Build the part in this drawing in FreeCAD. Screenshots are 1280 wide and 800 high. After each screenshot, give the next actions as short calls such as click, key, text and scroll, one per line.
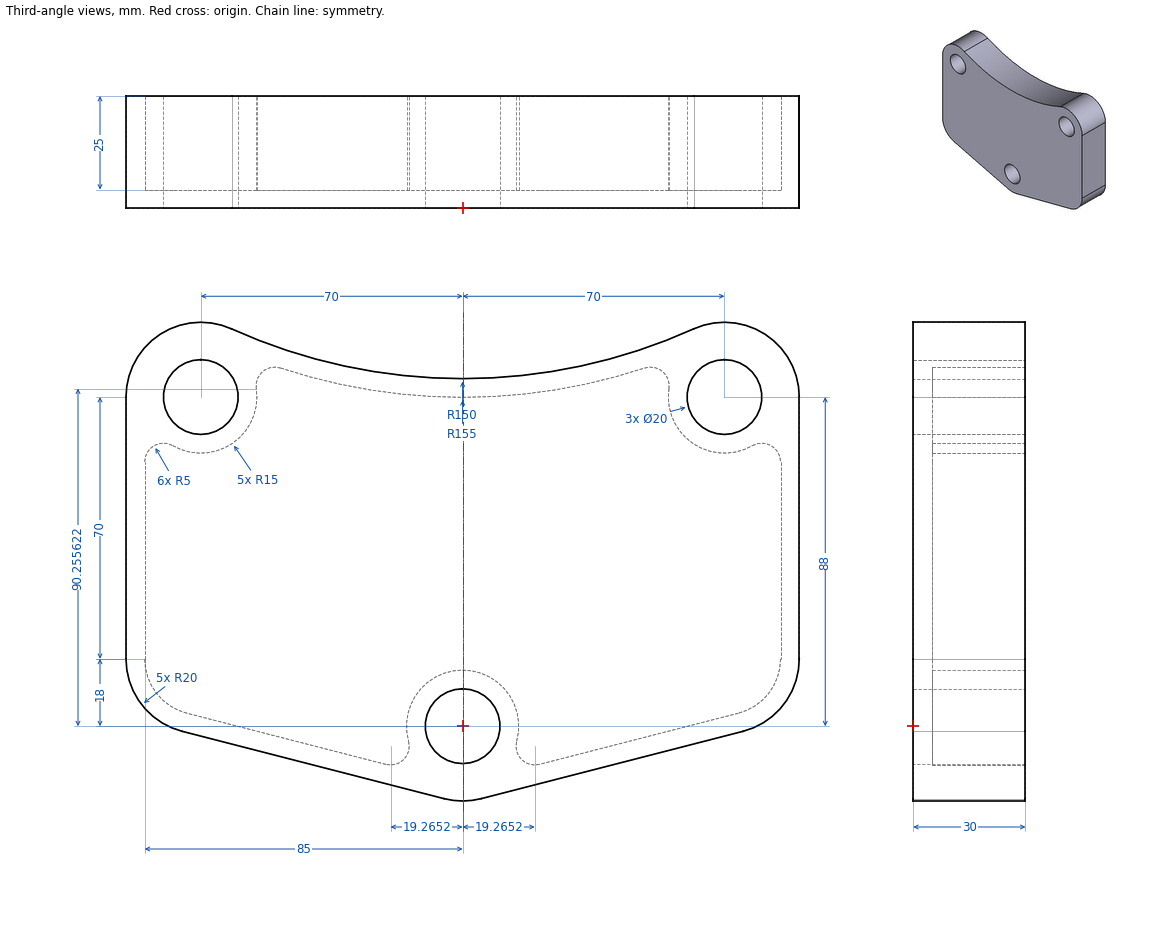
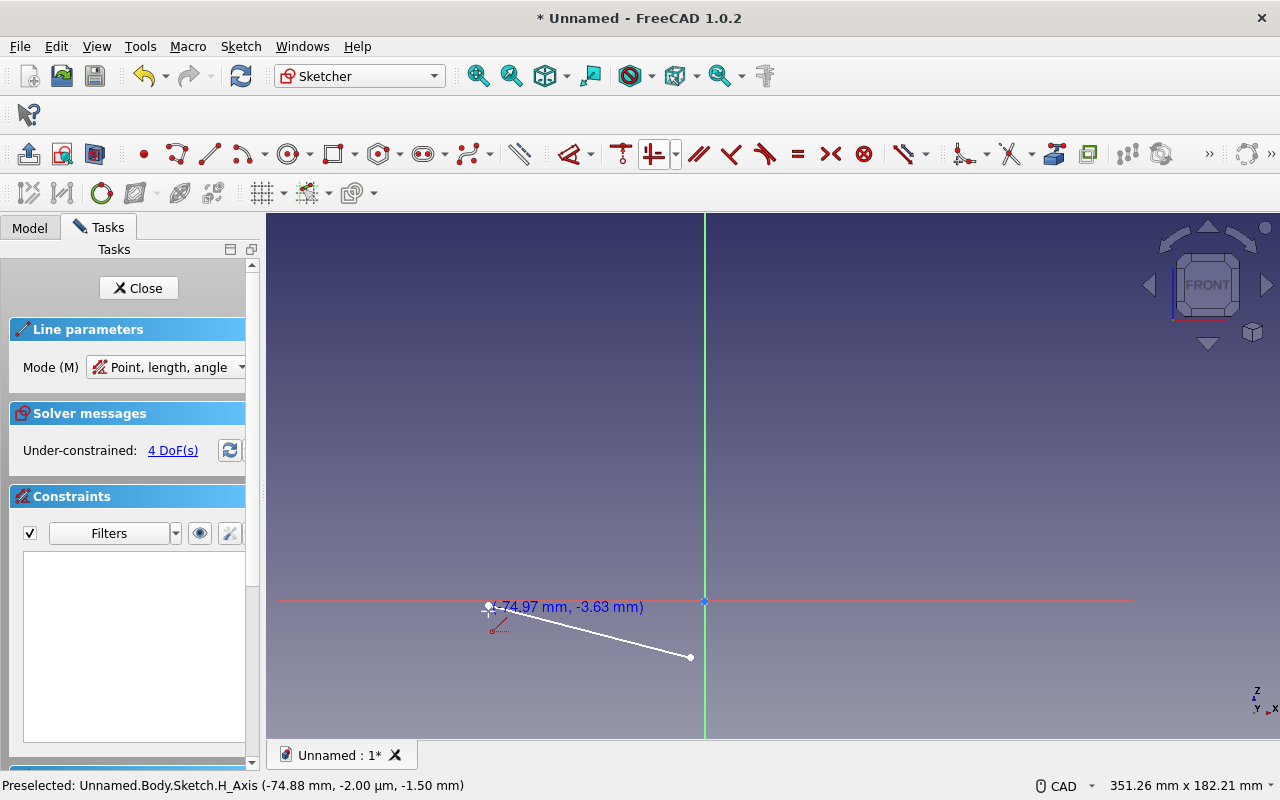
click(445, 549)
click(445, 347)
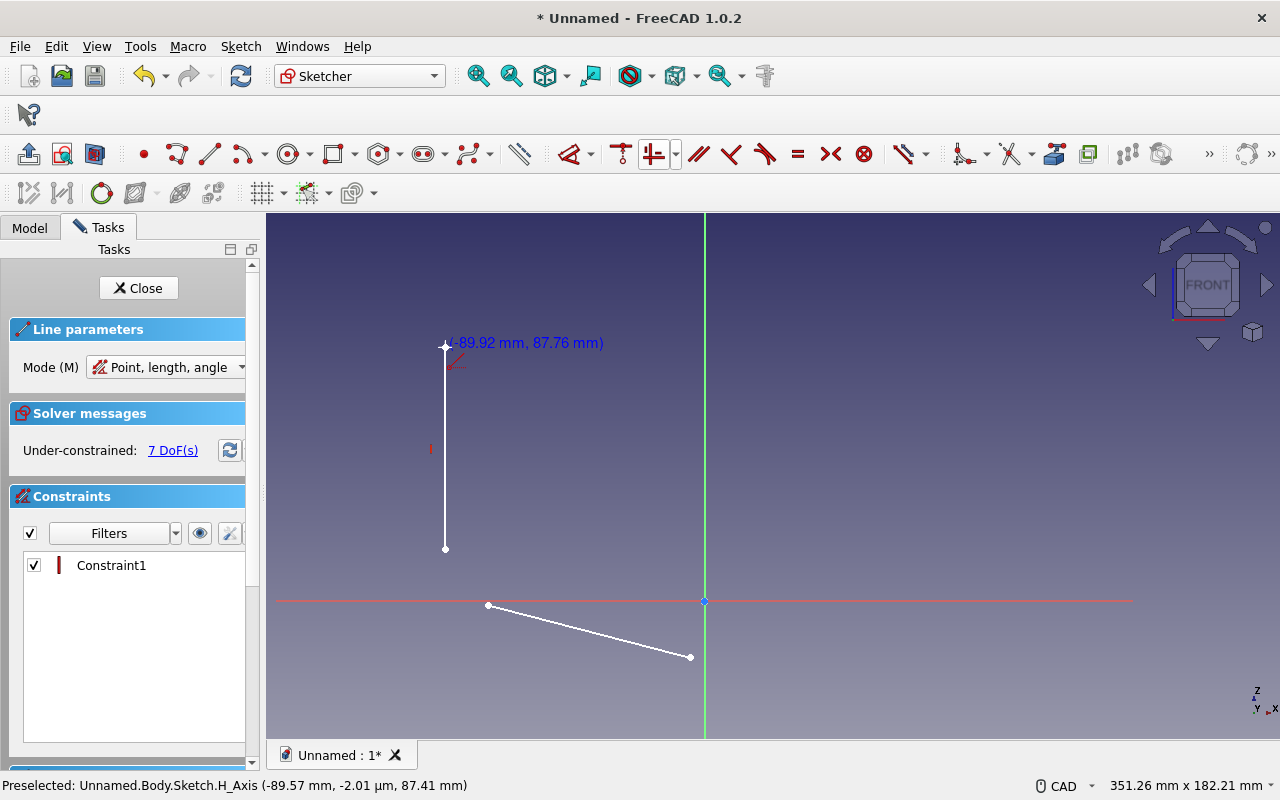
click(964, 347)
click(964, 549)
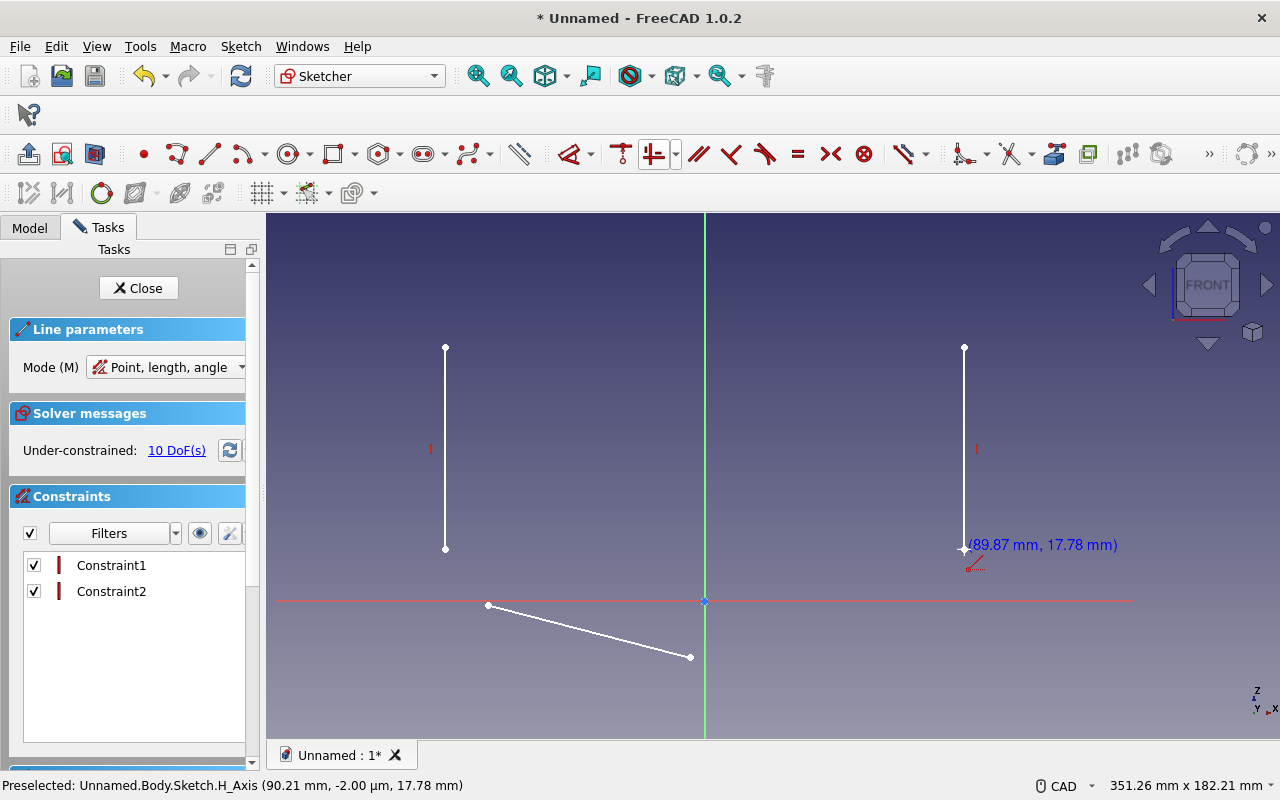
scroll(921, 605, up, 7)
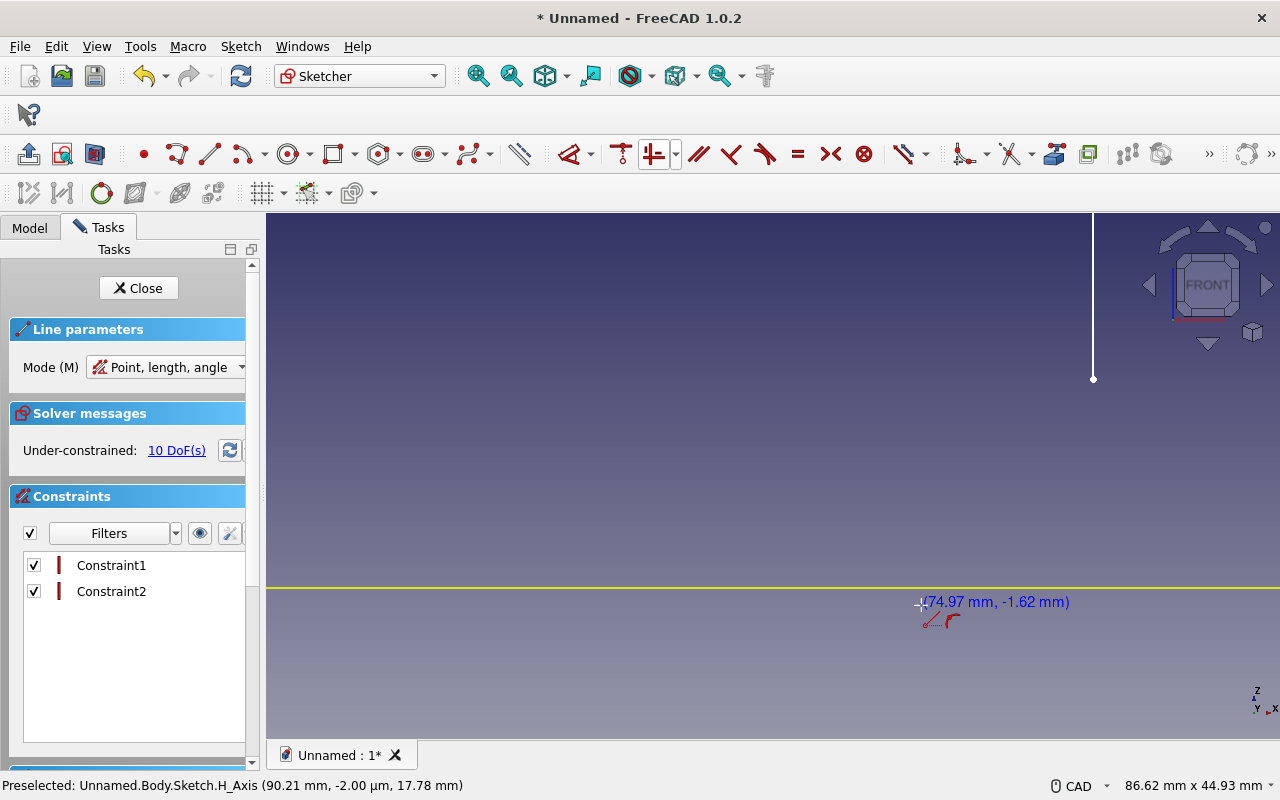
click(919, 604)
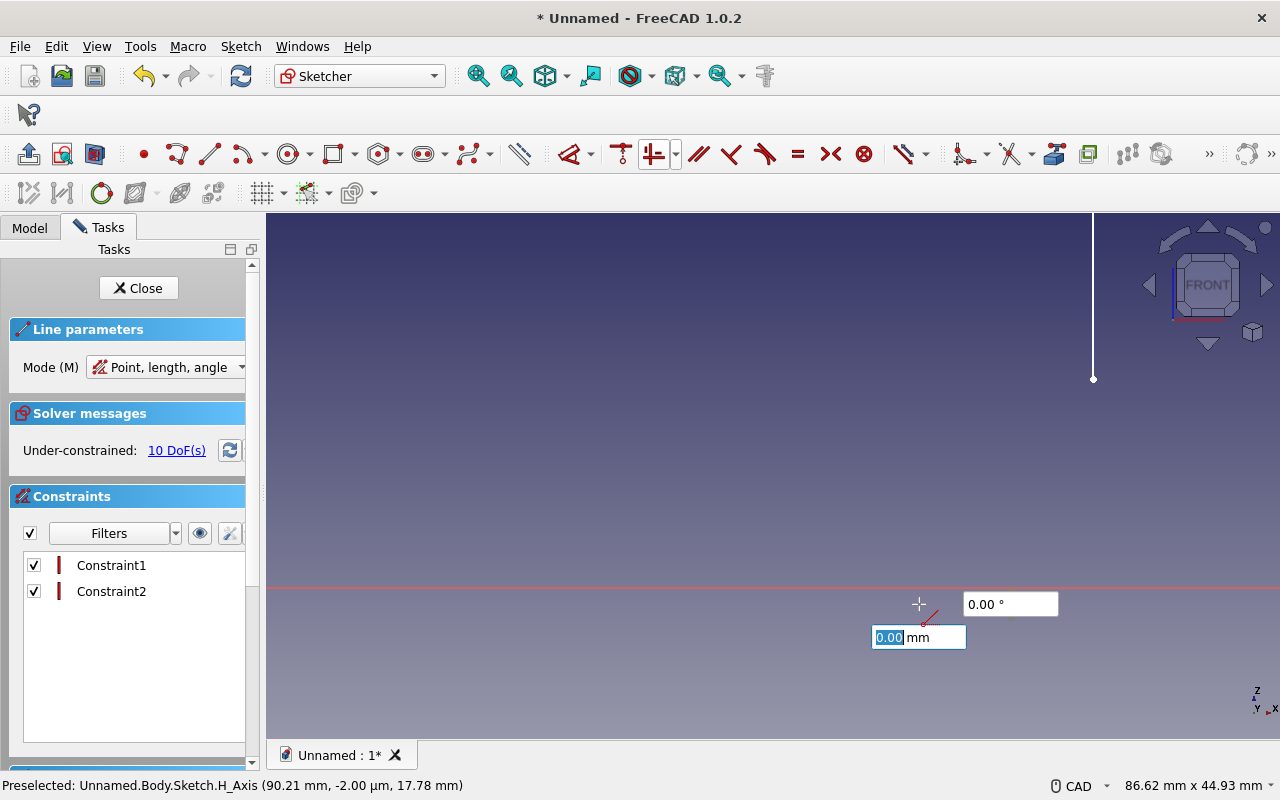
scroll(922, 605, down, 7)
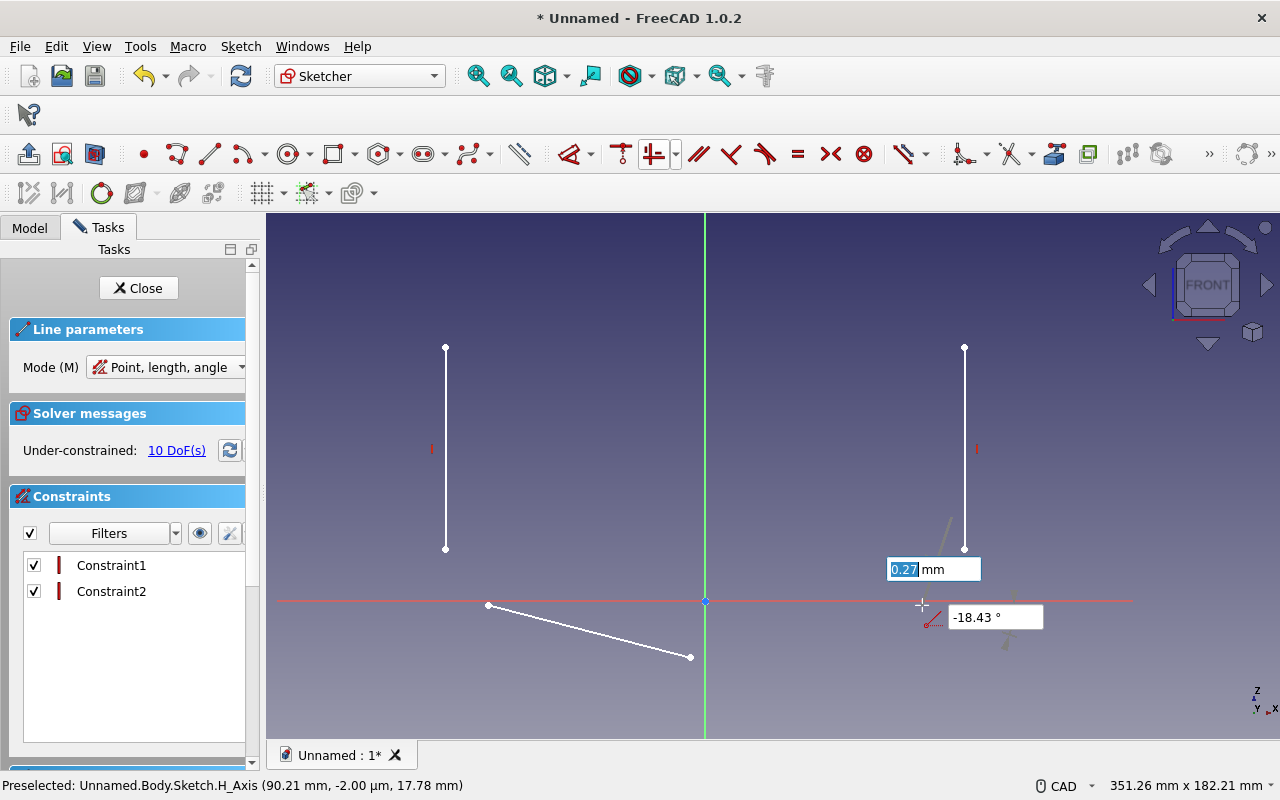
click(720, 657)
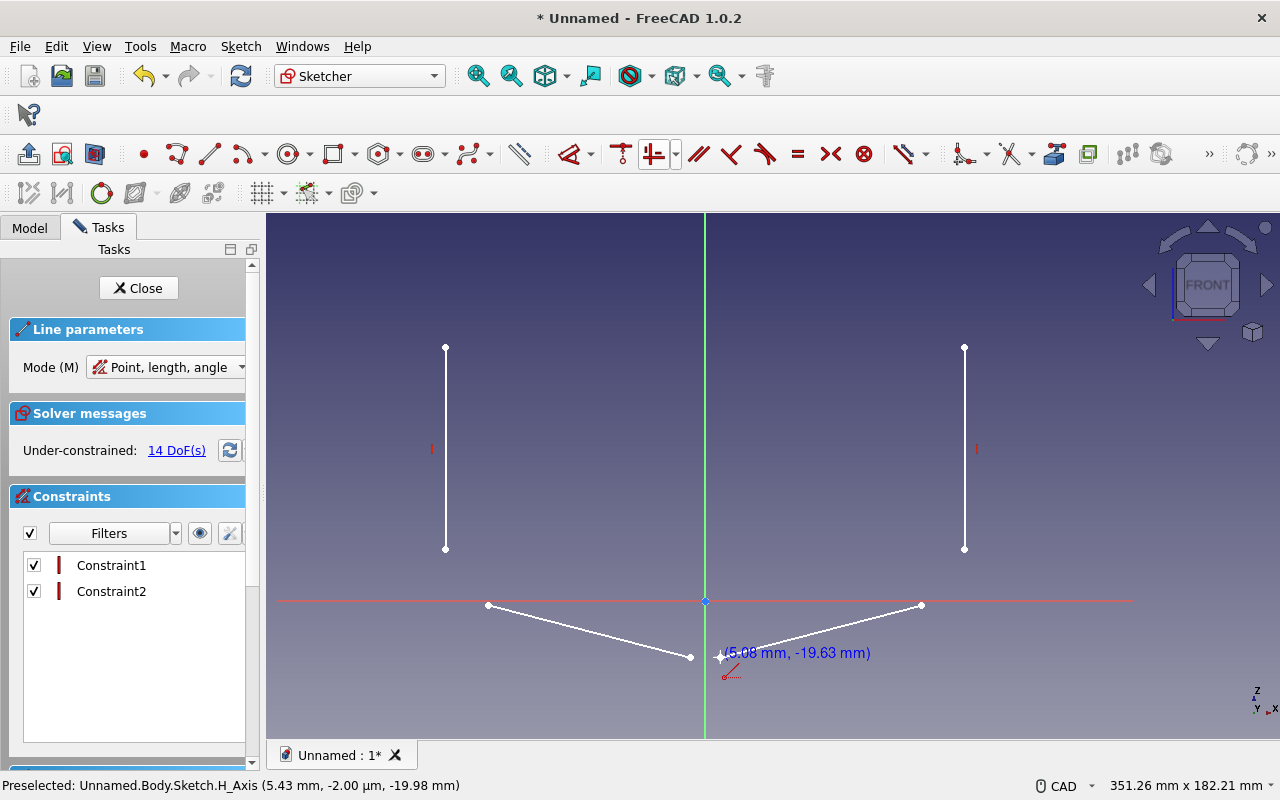
key(g)
key(3)
key(a)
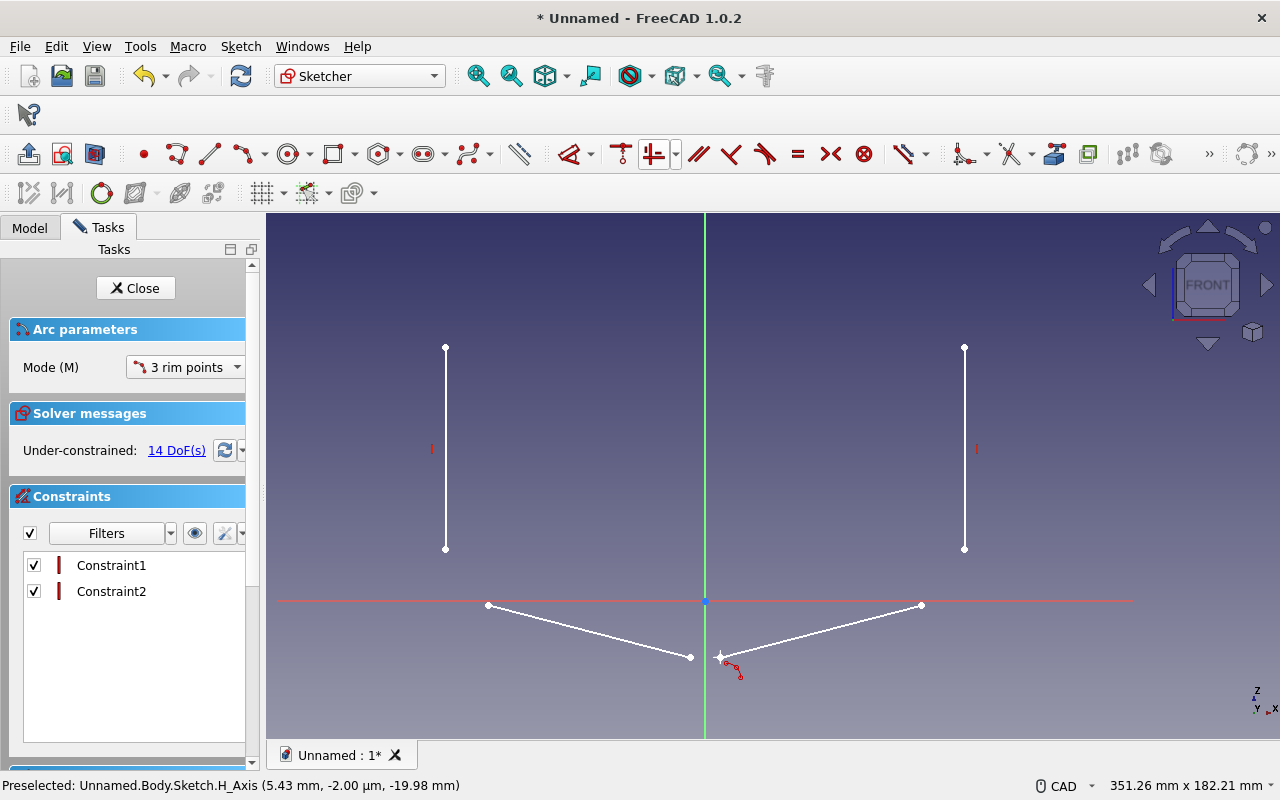
scroll(489, 605, up, 7)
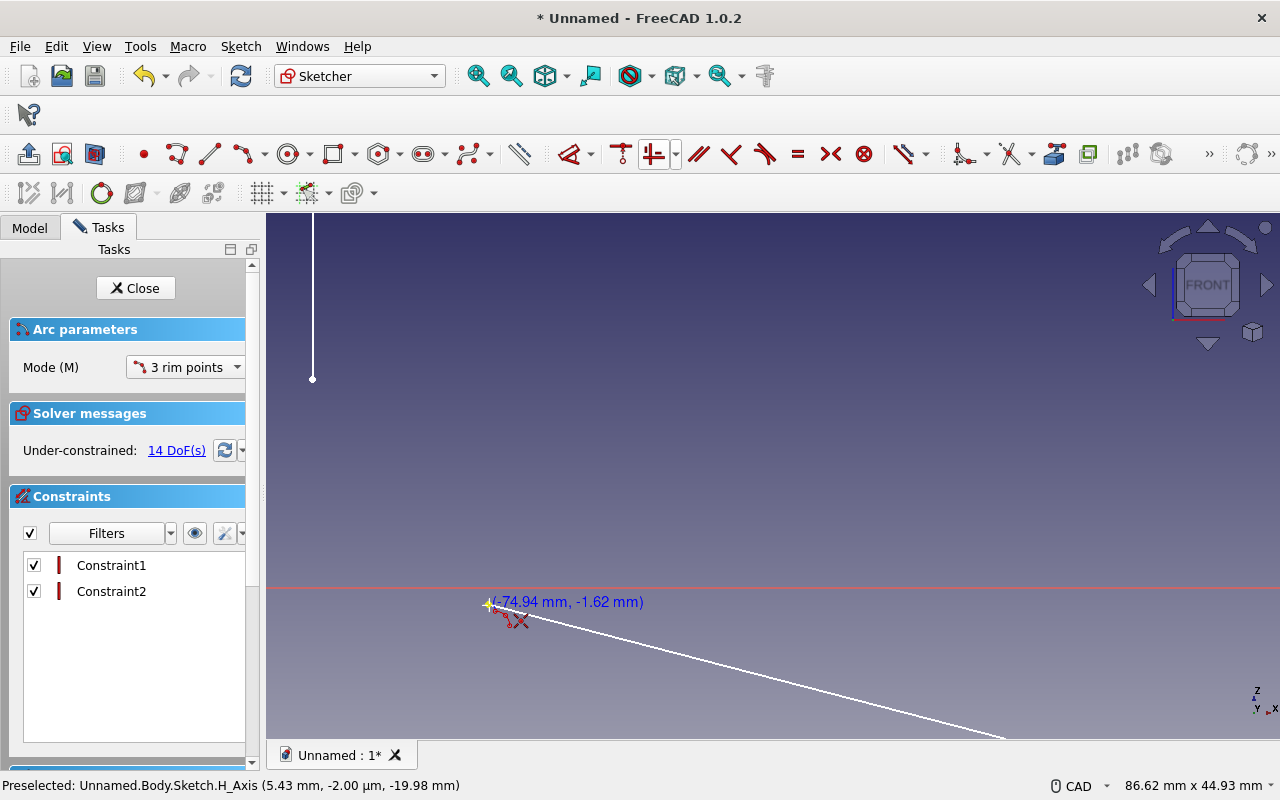
click(488, 604)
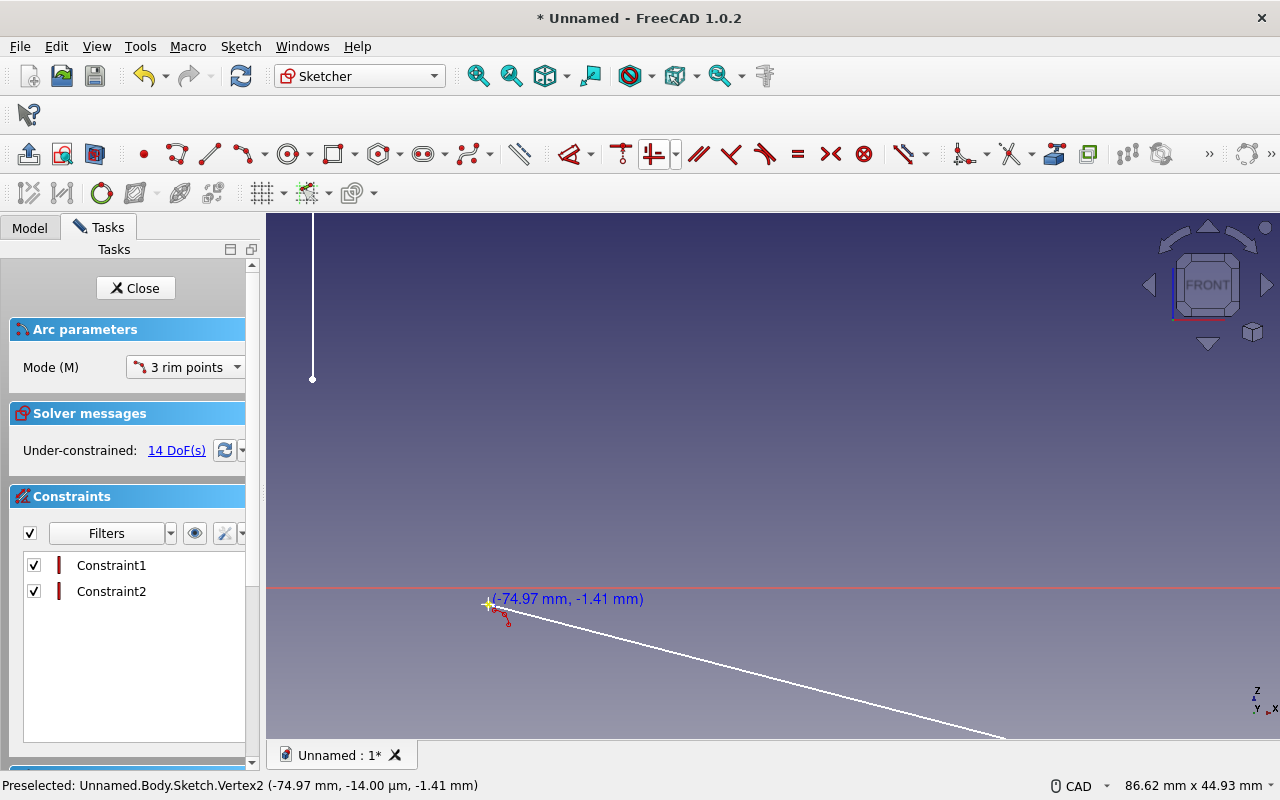
scroll(488, 605, down, 7)